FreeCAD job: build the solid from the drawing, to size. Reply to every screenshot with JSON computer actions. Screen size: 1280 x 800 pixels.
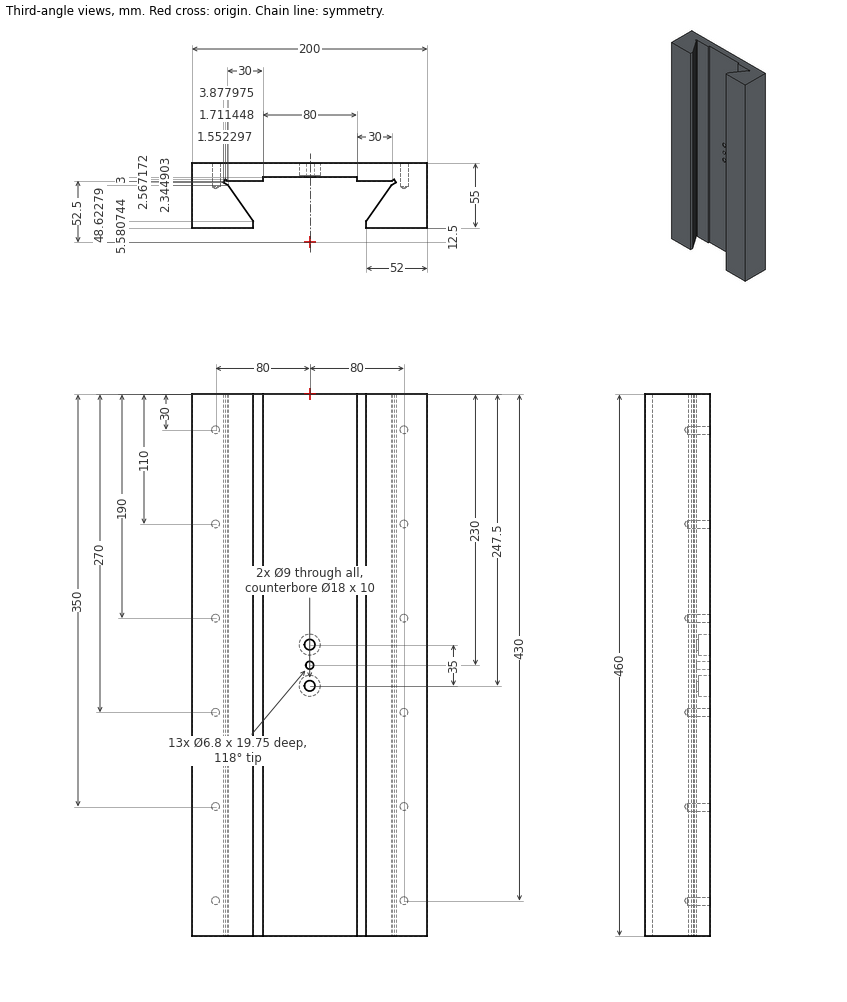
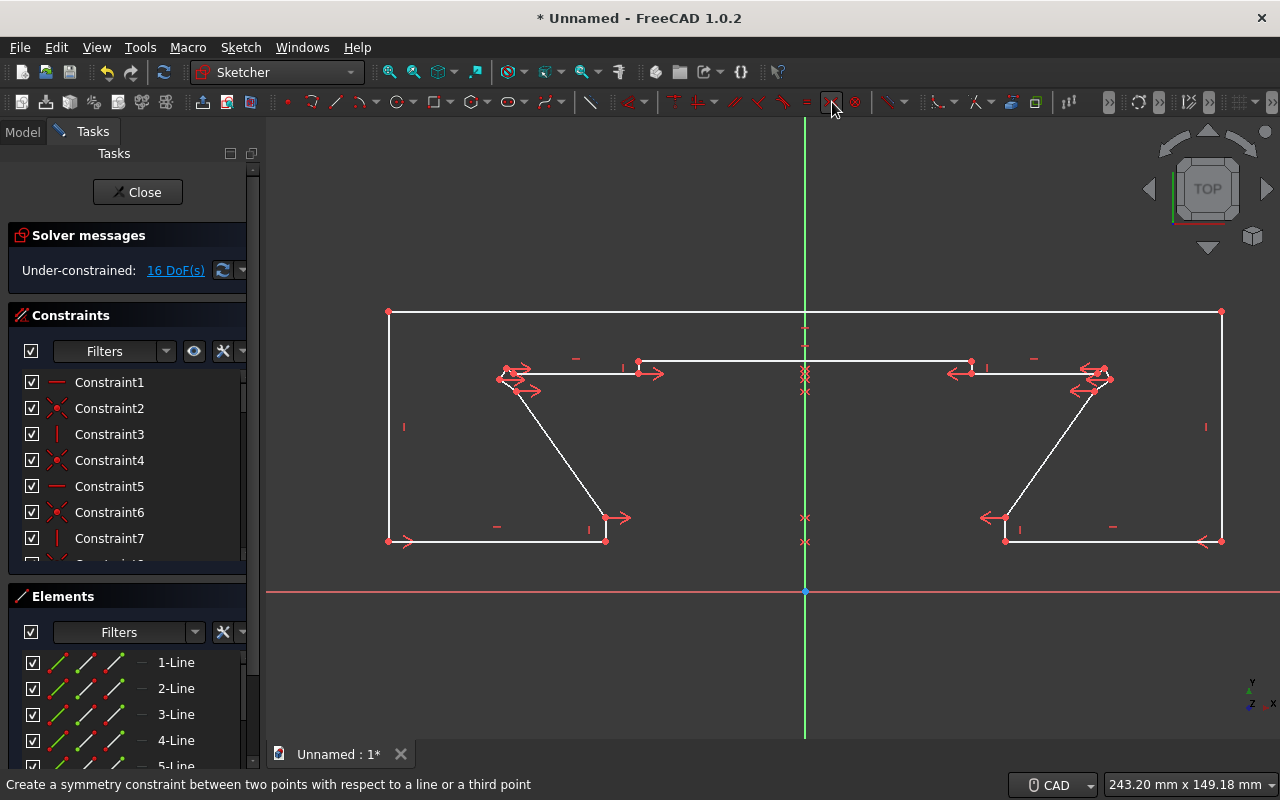
{"action": "left_click", "coordinate": [628, 102]}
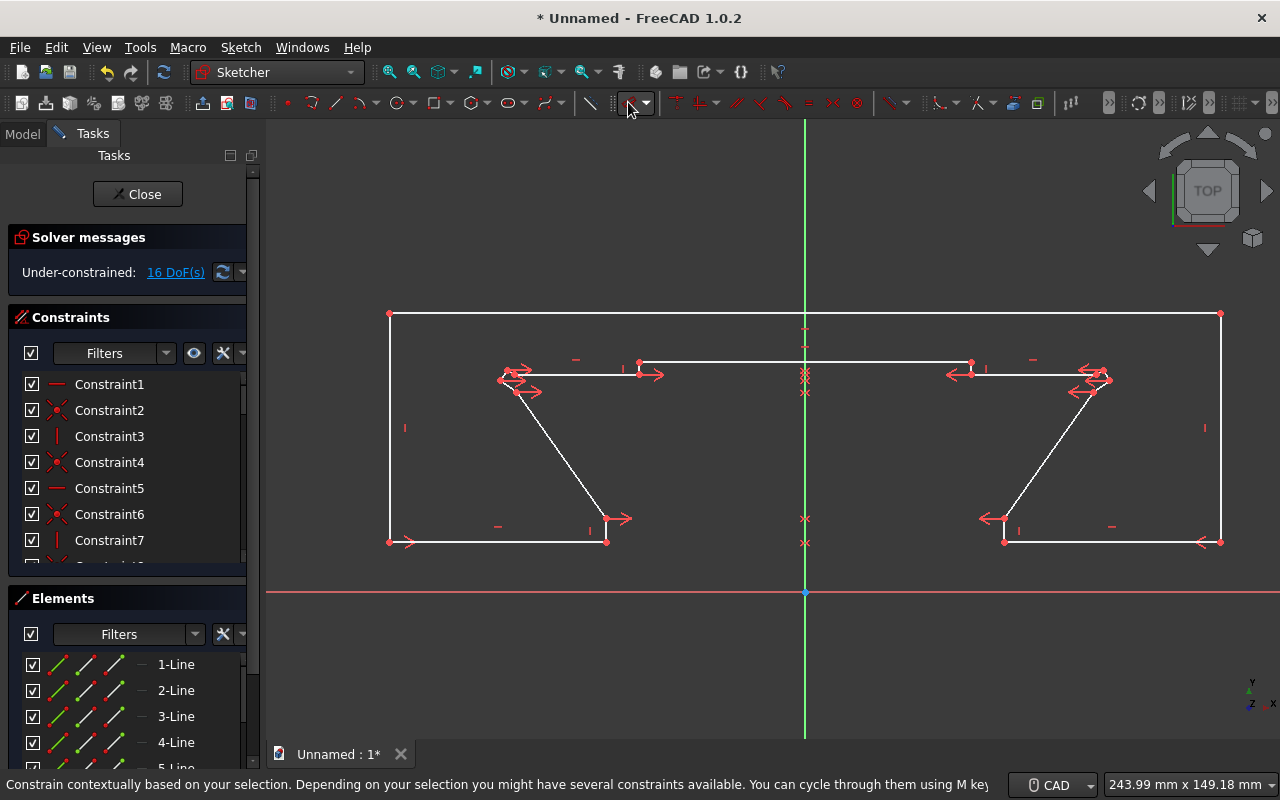
{"action": "scroll", "coordinate": [639, 369], "scroll_direction": "up", "scroll_amount": 6}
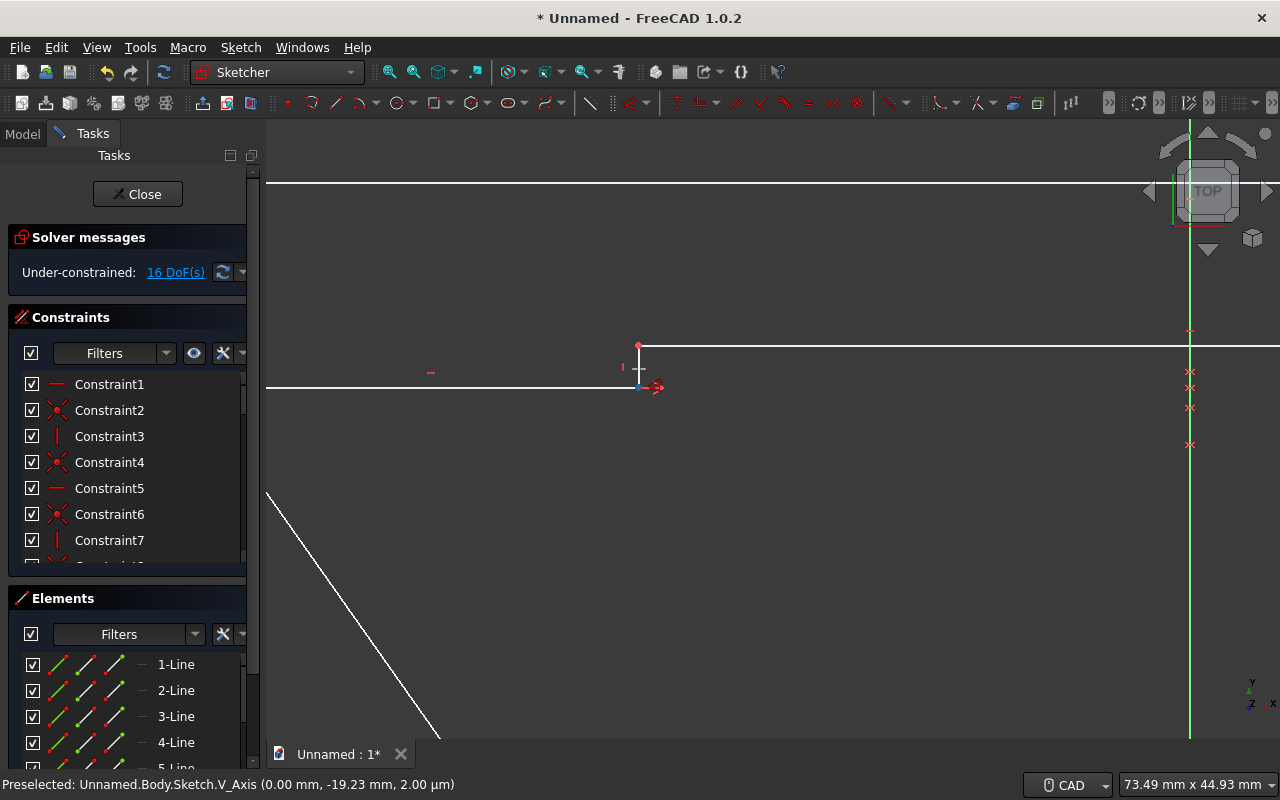
{"action": "left_click", "coordinate": [639, 367]}
{"action": "left_click", "coordinate": [605, 367]}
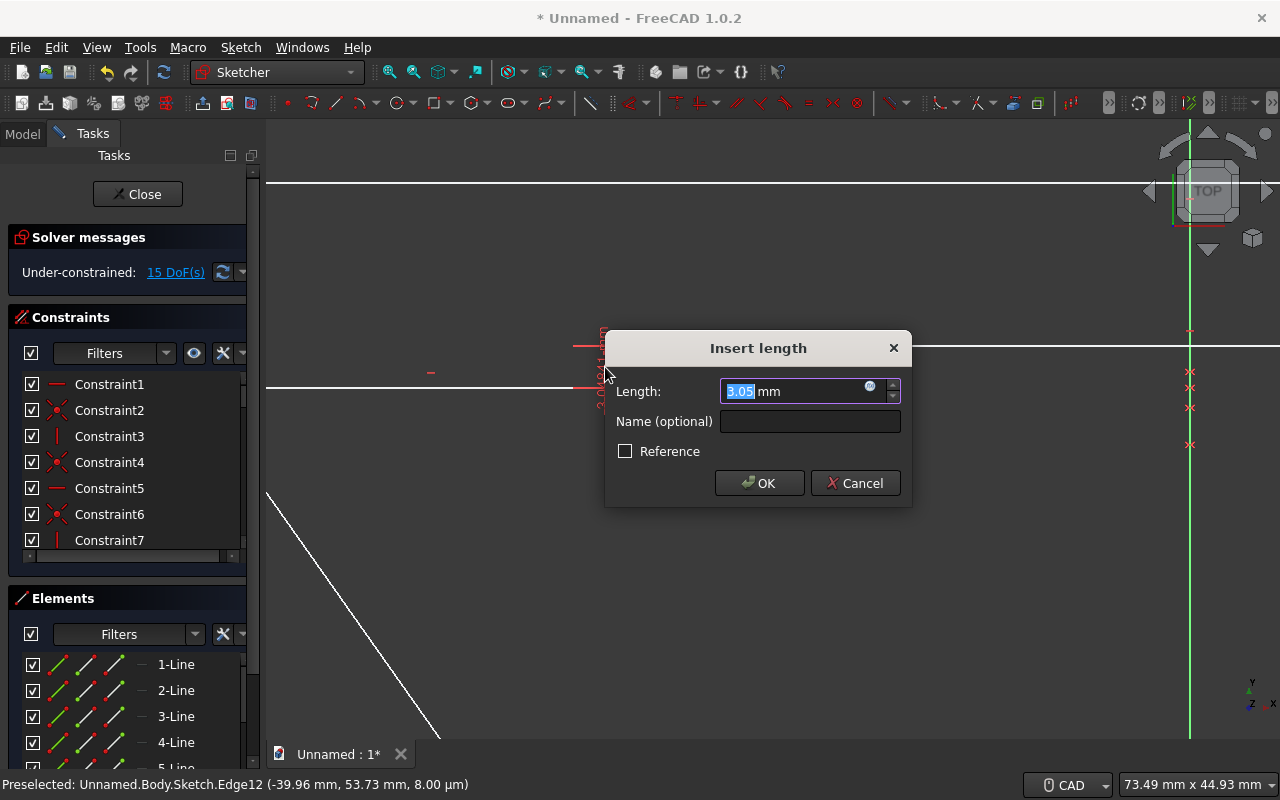
{"action": "type", "text": "3"}
{"action": "key", "text": "Return"}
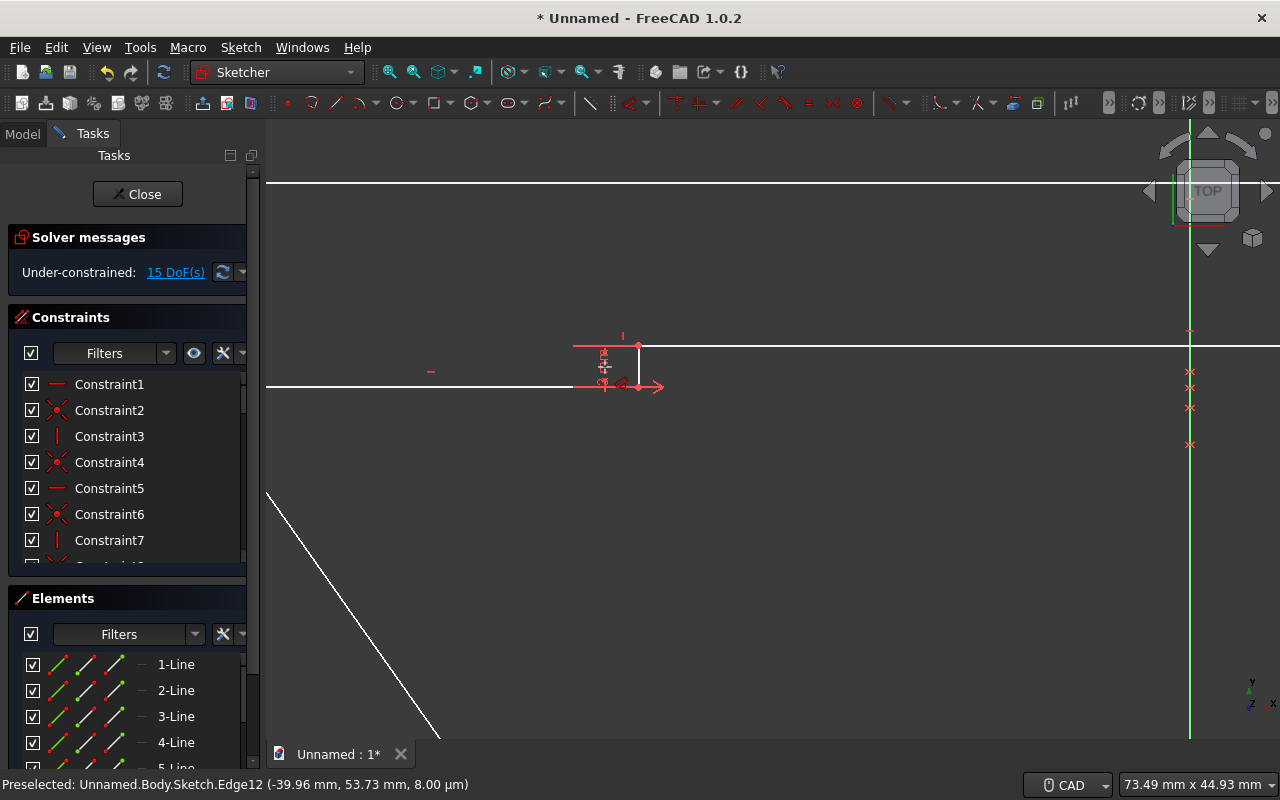
{"action": "scroll", "coordinate": [582, 375], "scroll_direction": "down", "scroll_amount": 8}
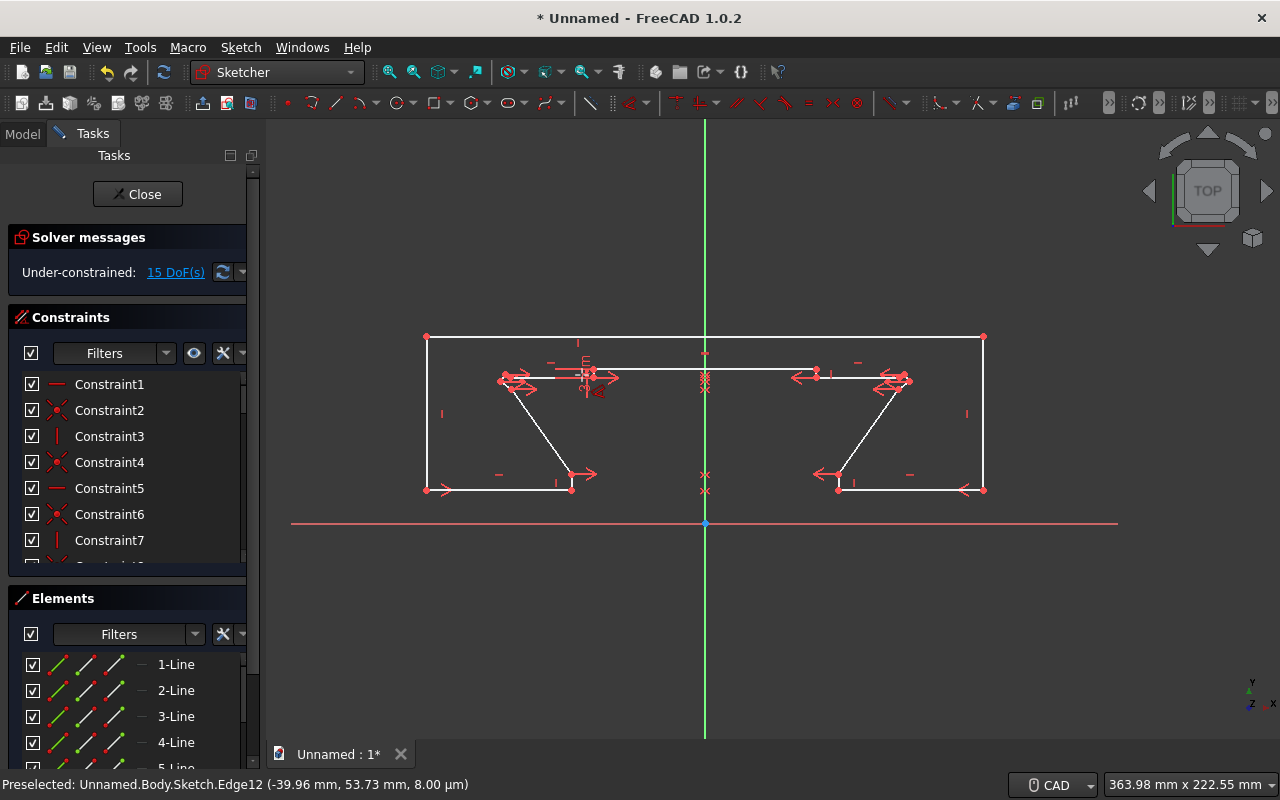
{"action": "left_click", "coordinate": [882, 490]}
{"action": "left_click", "coordinate": [911, 456]}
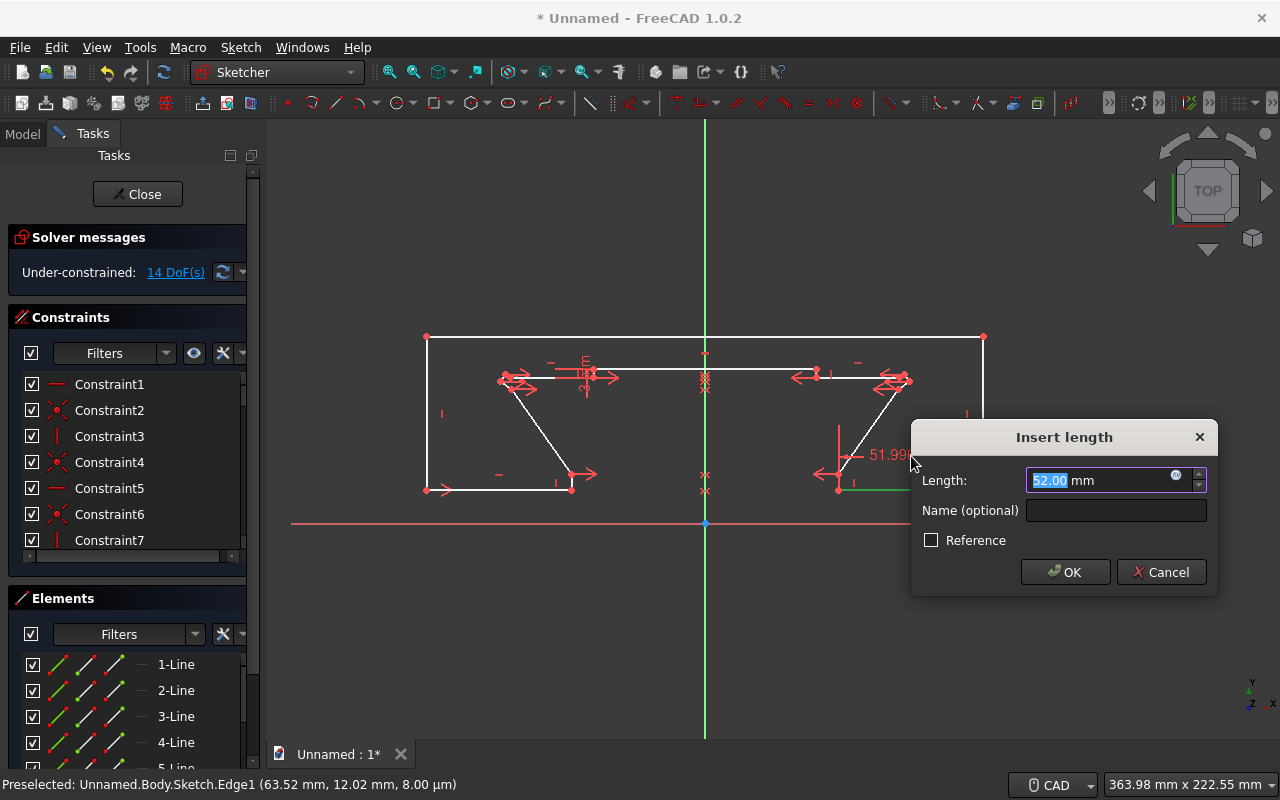
{"action": "type", "text": "52"}
{"action": "key", "text": "Return"}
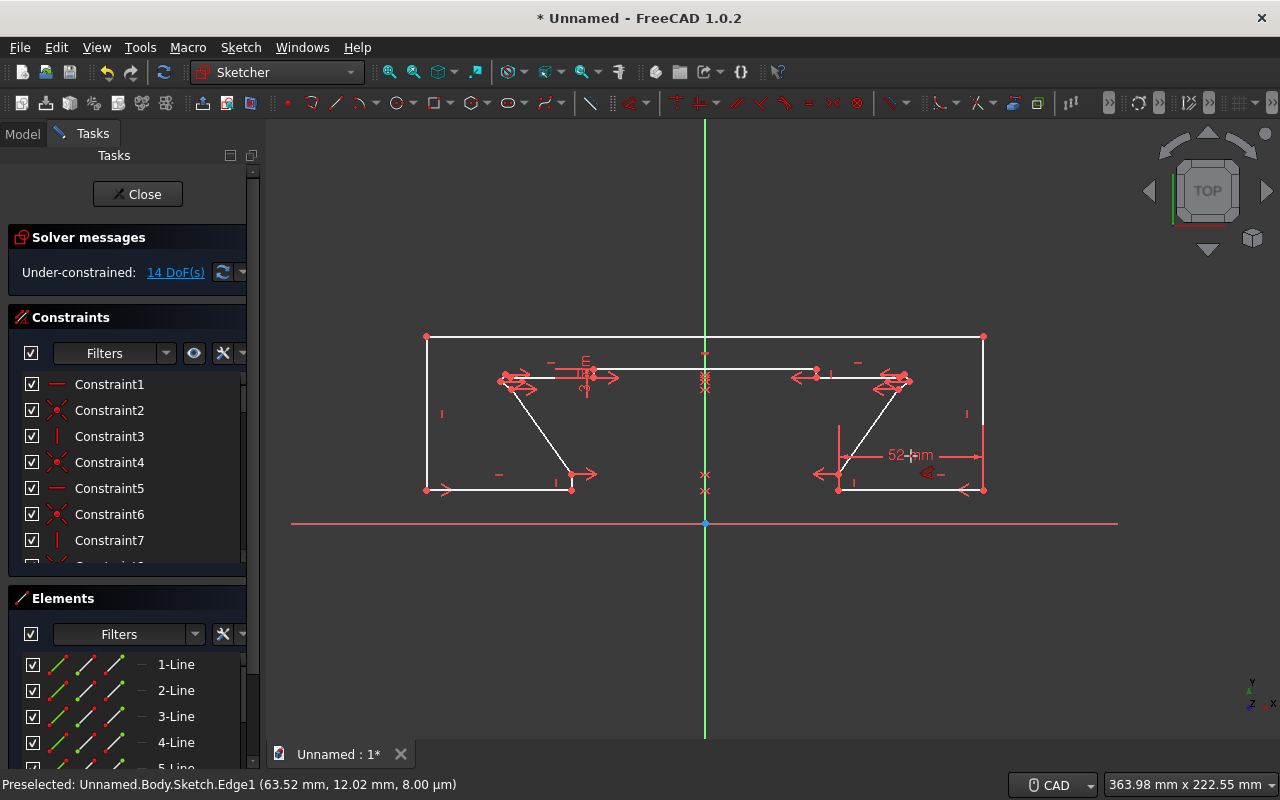
{"action": "left_click", "coordinate": [983, 444]}
{"action": "left_click", "coordinate": [1017, 413]}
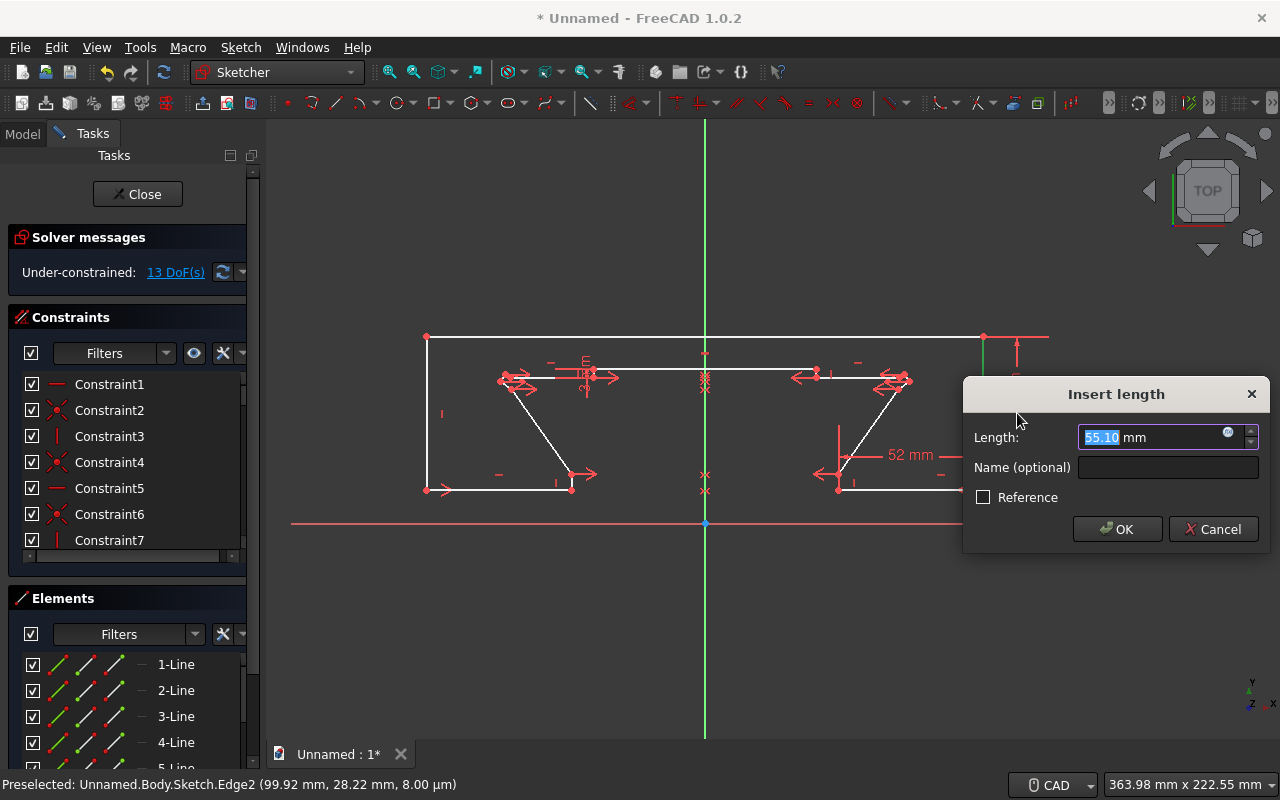
{"action": "type", "text": "55"}
{"action": "key", "text": "Return"}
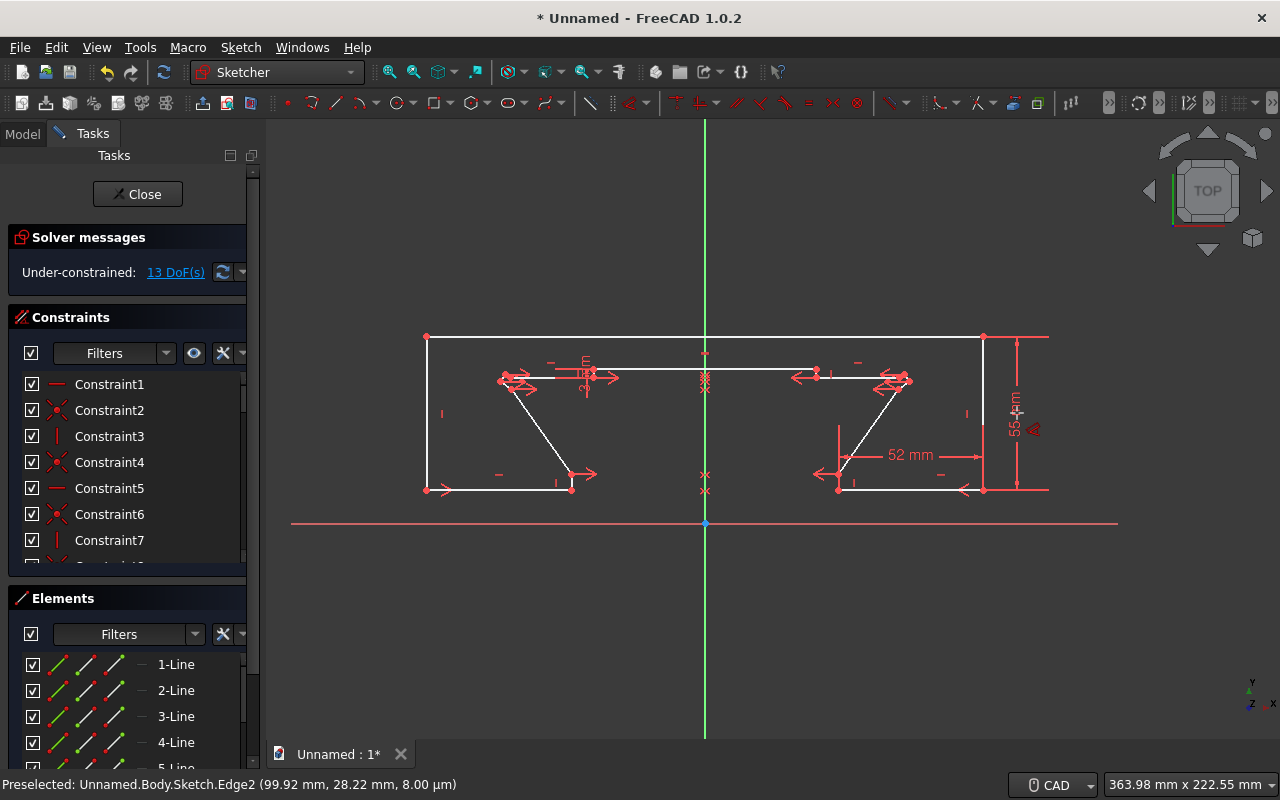
{"action": "left_click", "coordinate": [535, 378]}
{"action": "left_click", "coordinate": [552, 412]}